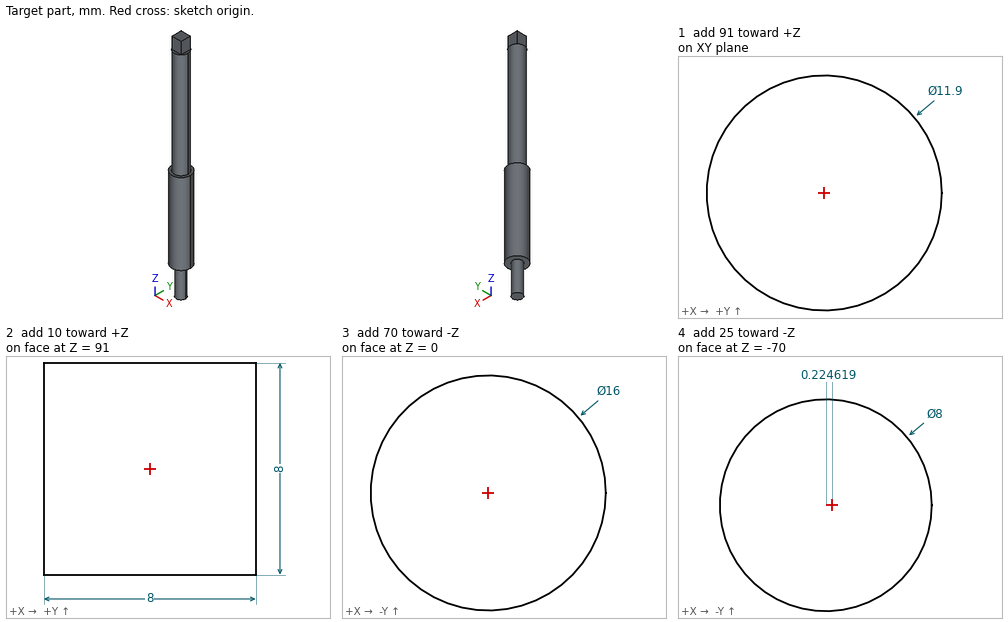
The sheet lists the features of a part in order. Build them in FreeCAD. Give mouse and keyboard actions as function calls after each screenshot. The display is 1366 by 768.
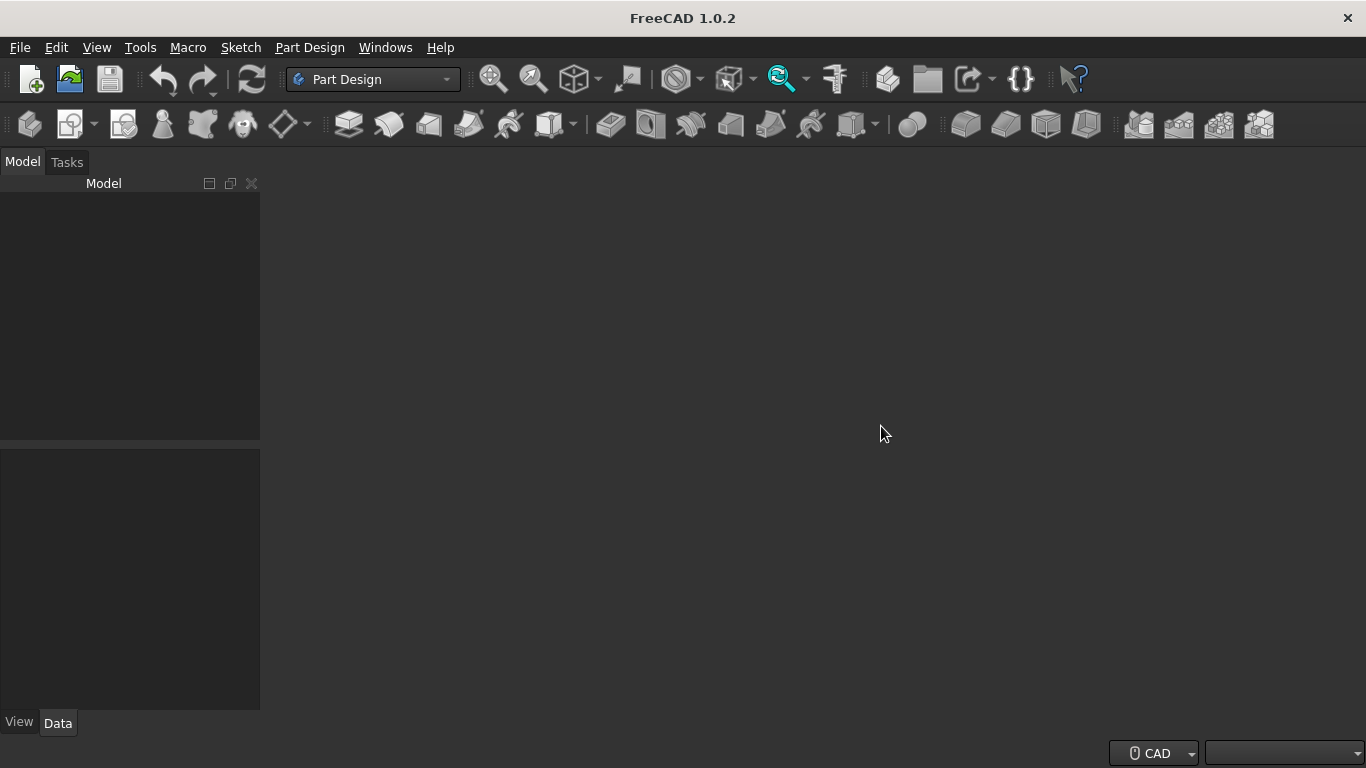
click(30, 80)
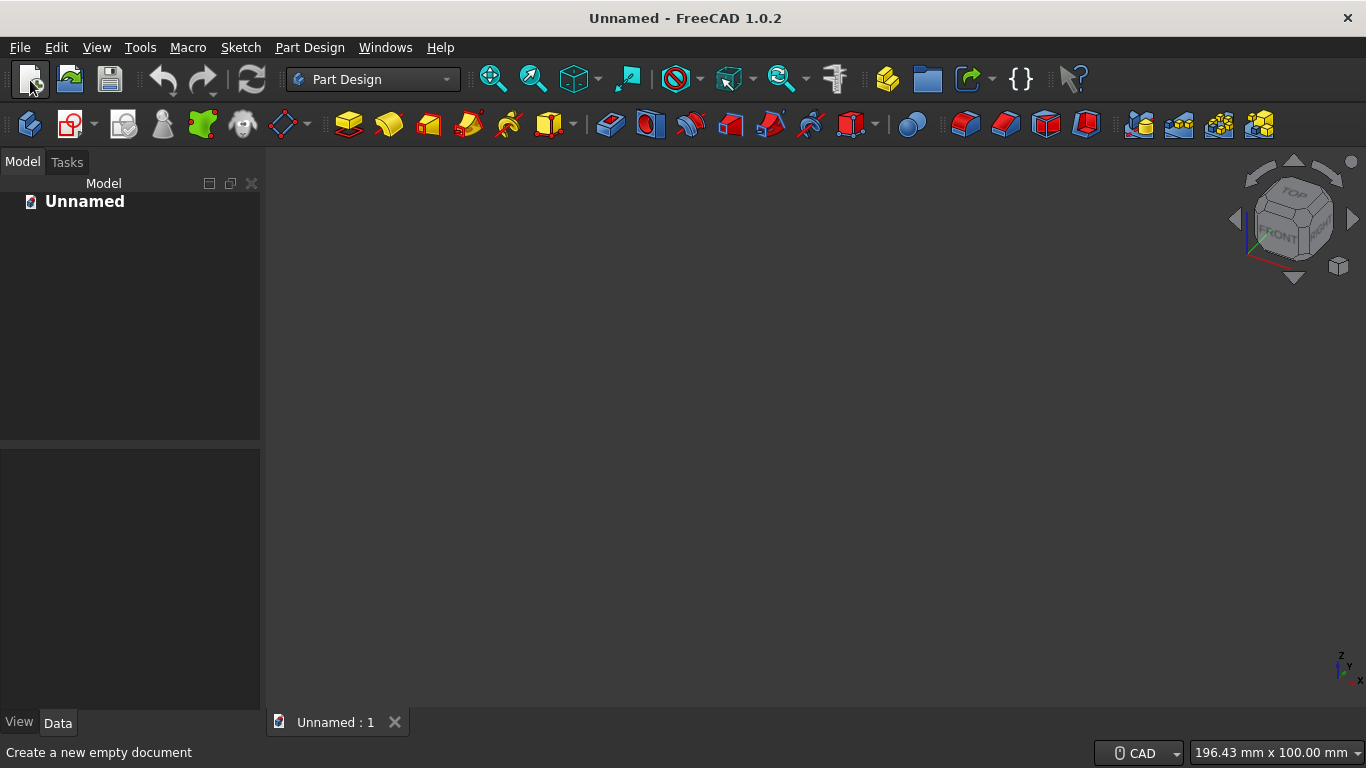
click(70, 124)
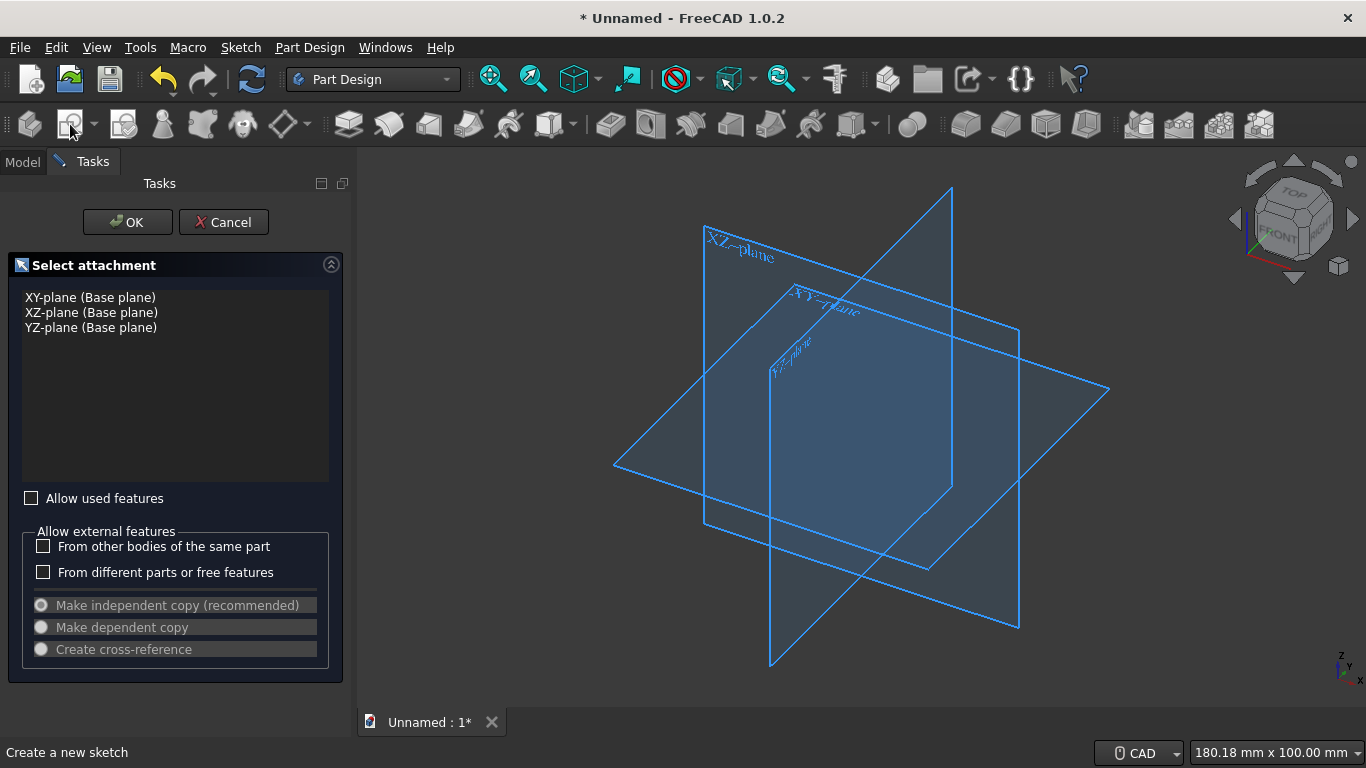
click(82, 298)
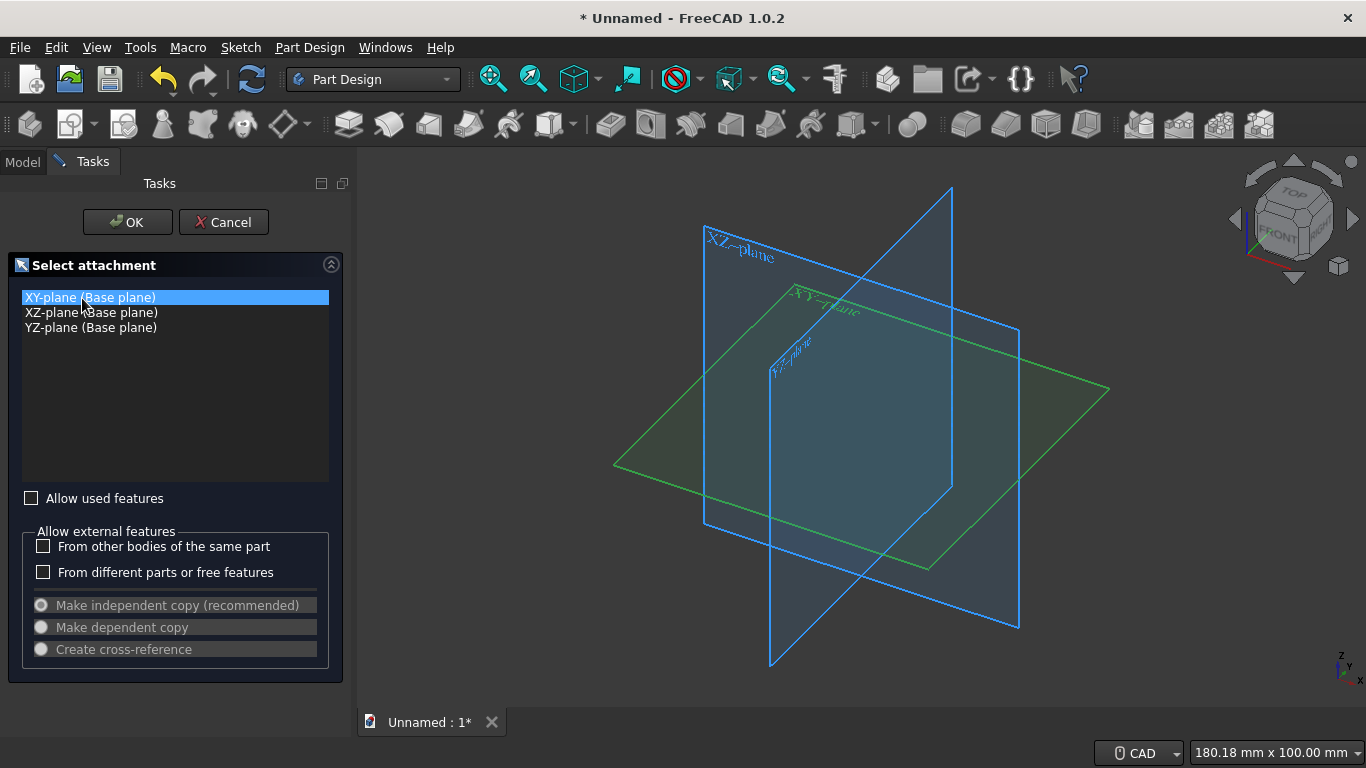
click(128, 222)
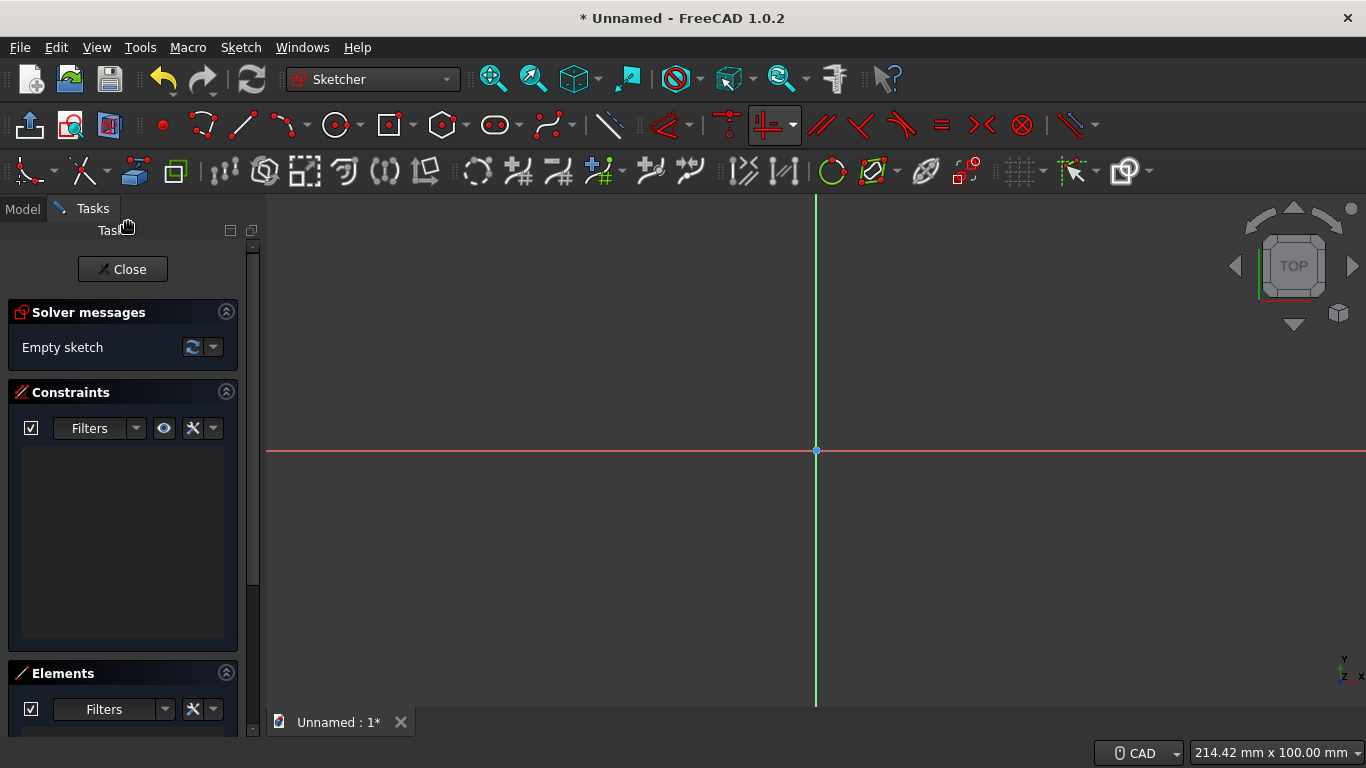
scroll(833, 450, up, 8)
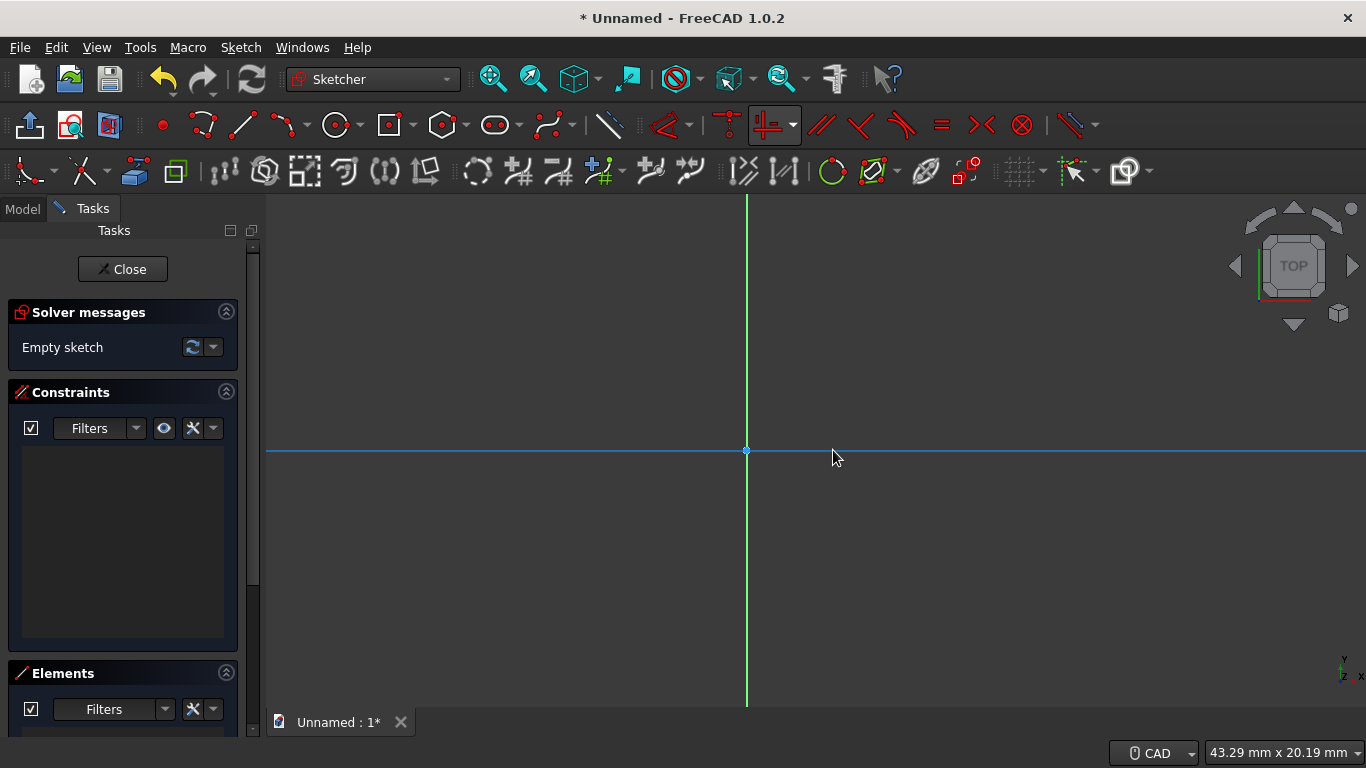
key(g)
key(c)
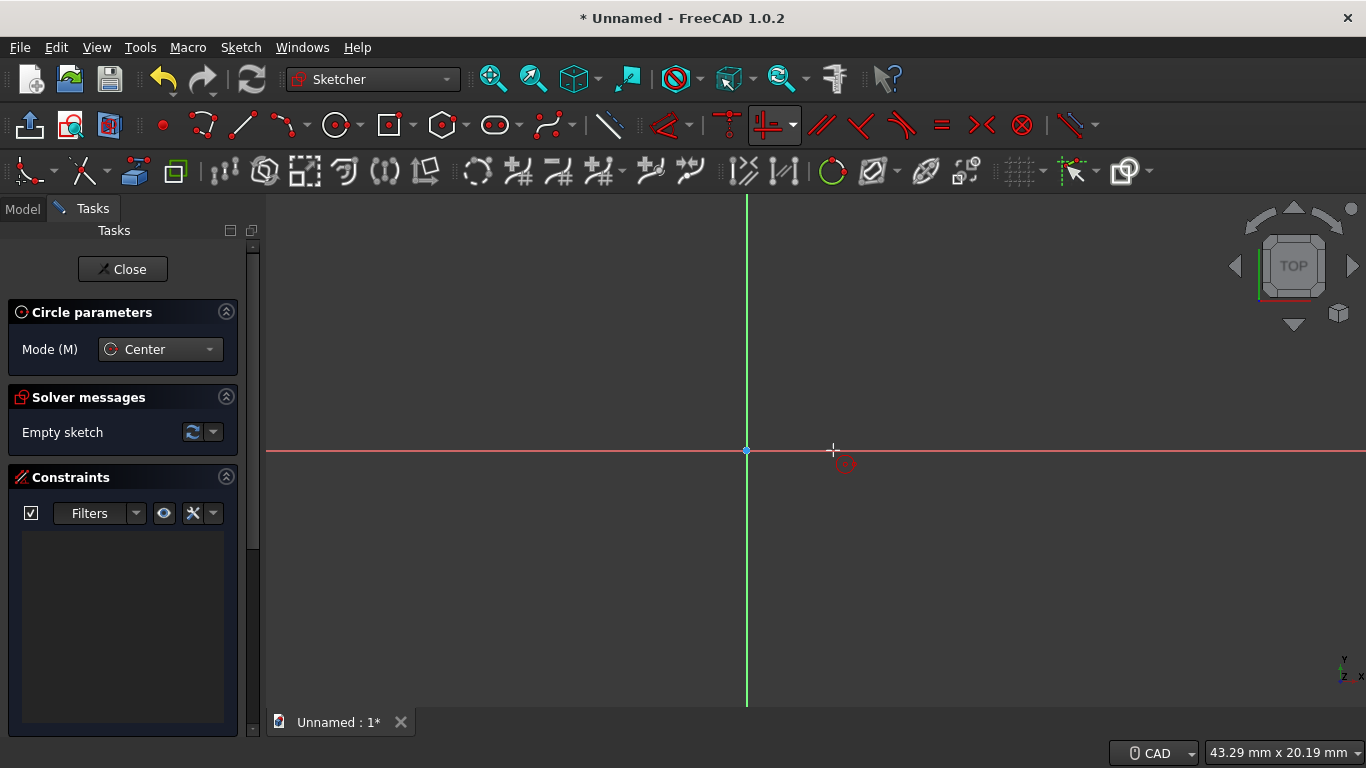
click(747, 450)
click(854, 344)
key(Escape)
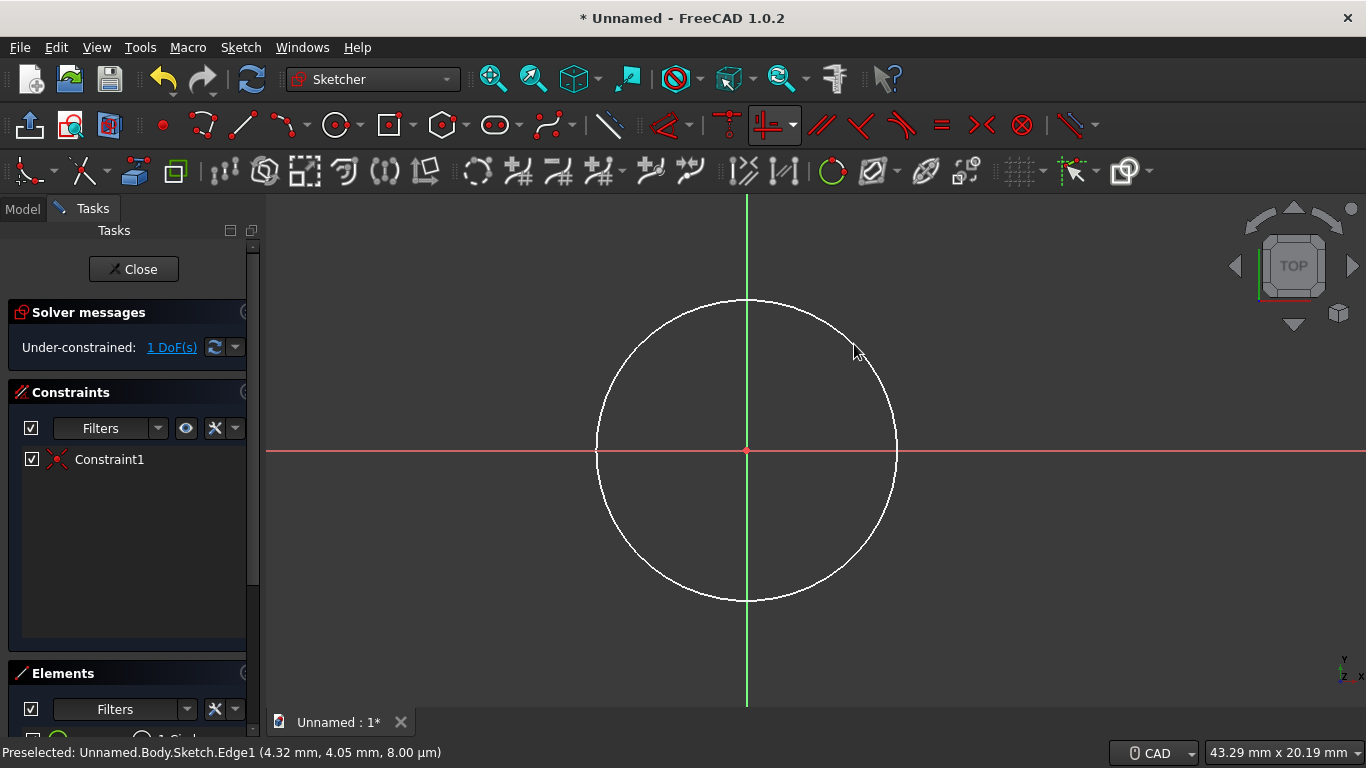
click(853, 344)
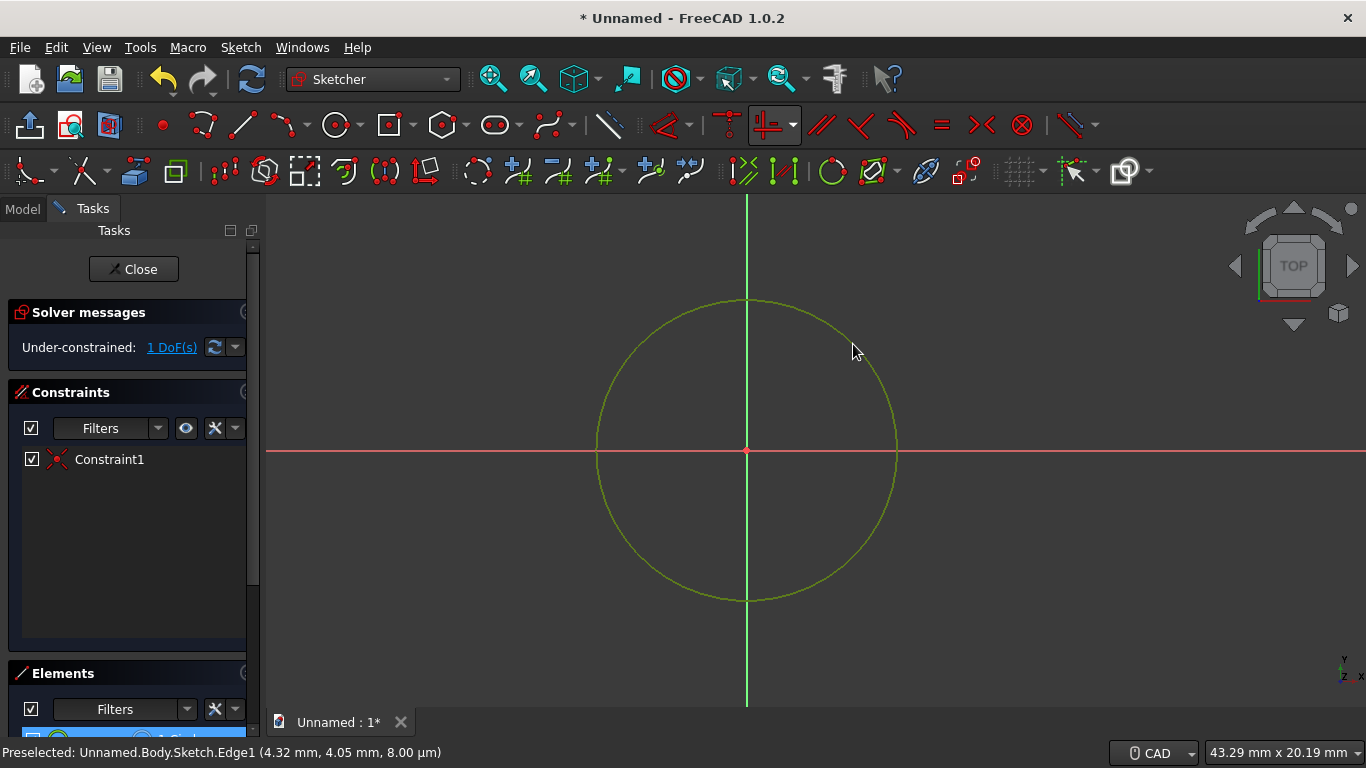
click(692, 126)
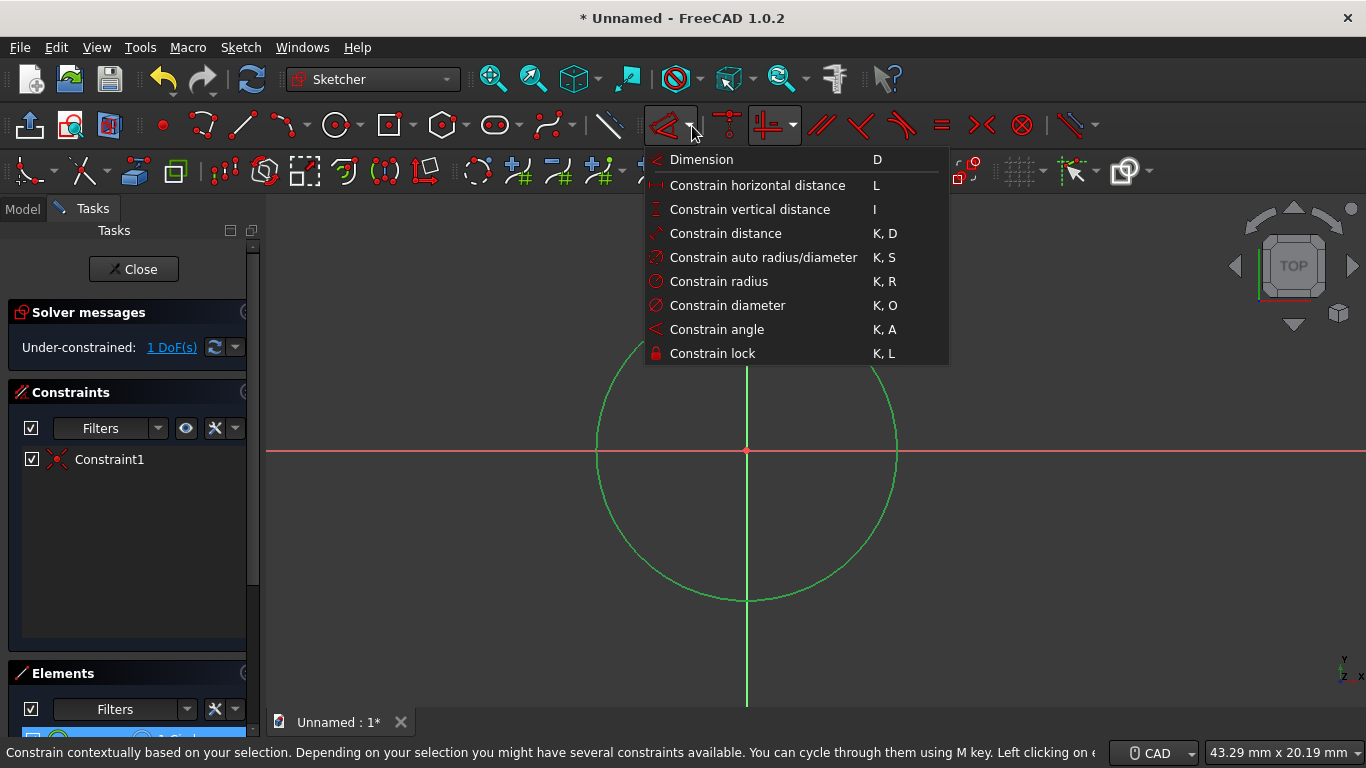
click(797, 305)